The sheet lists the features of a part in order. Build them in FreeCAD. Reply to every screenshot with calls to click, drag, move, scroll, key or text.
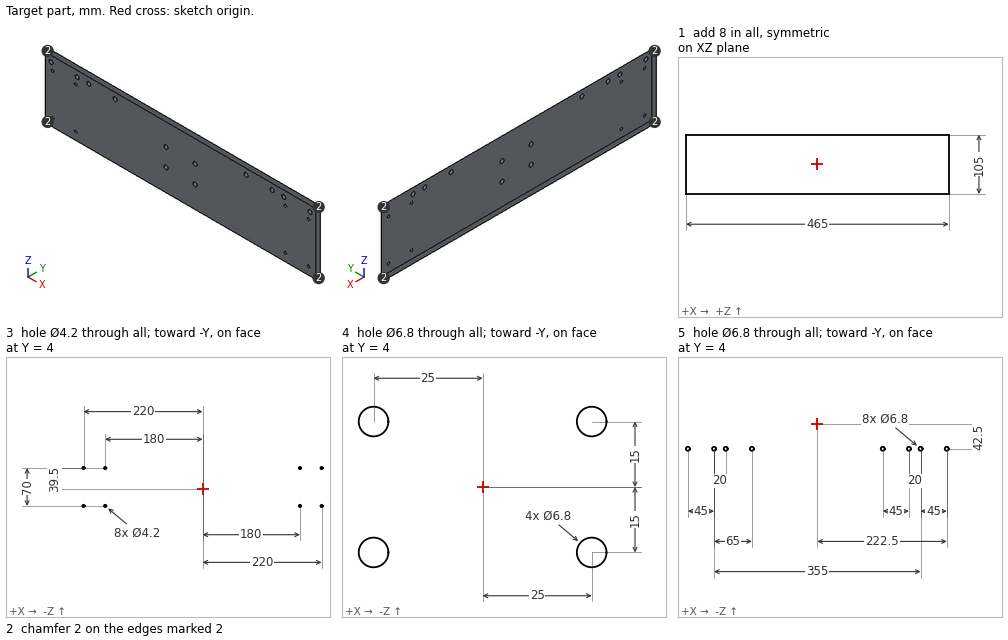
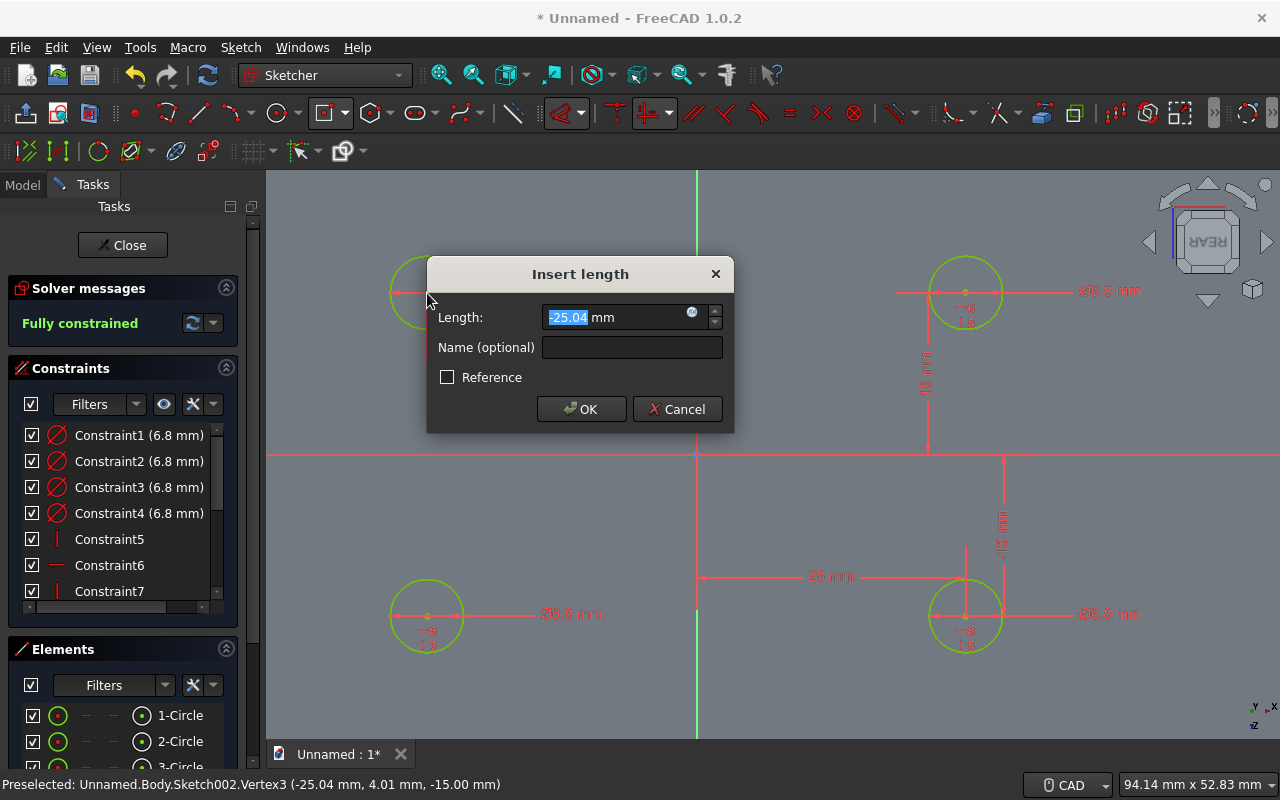
text(-25)
key(Return)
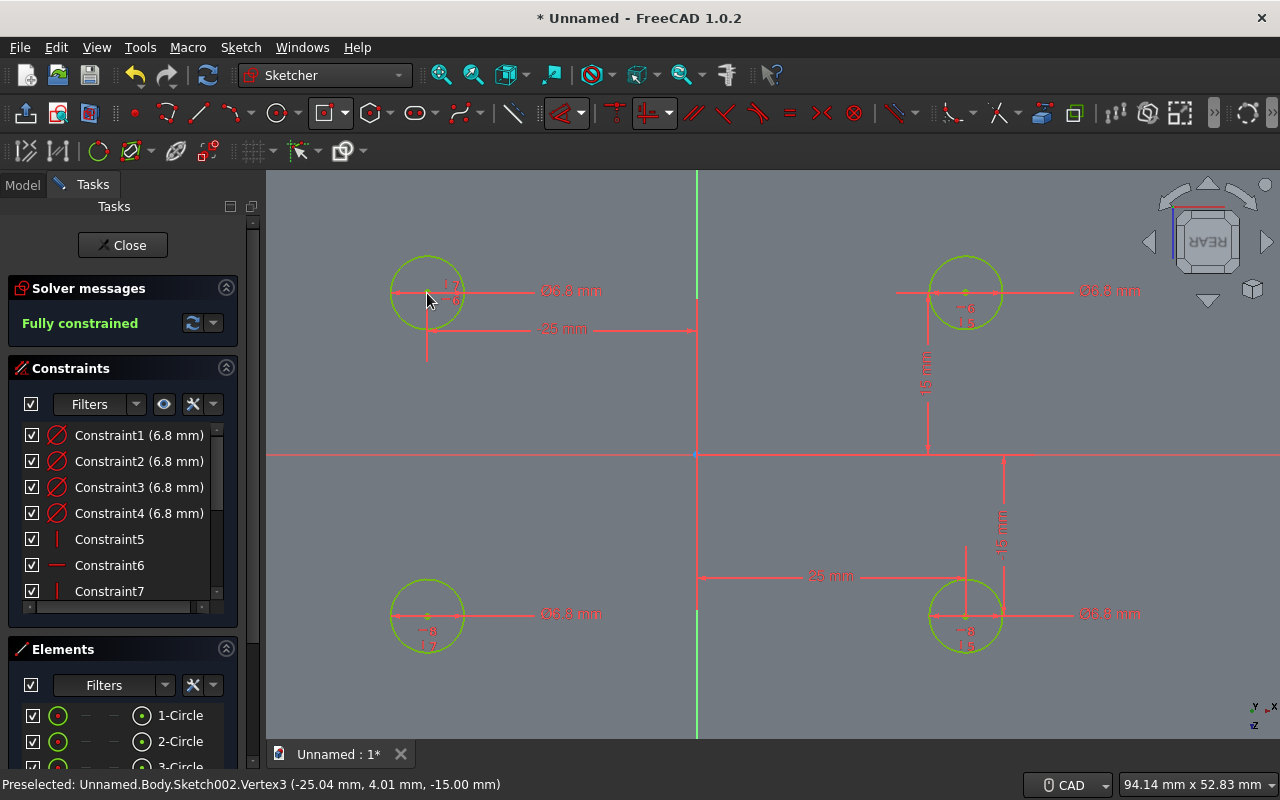
click(123, 245)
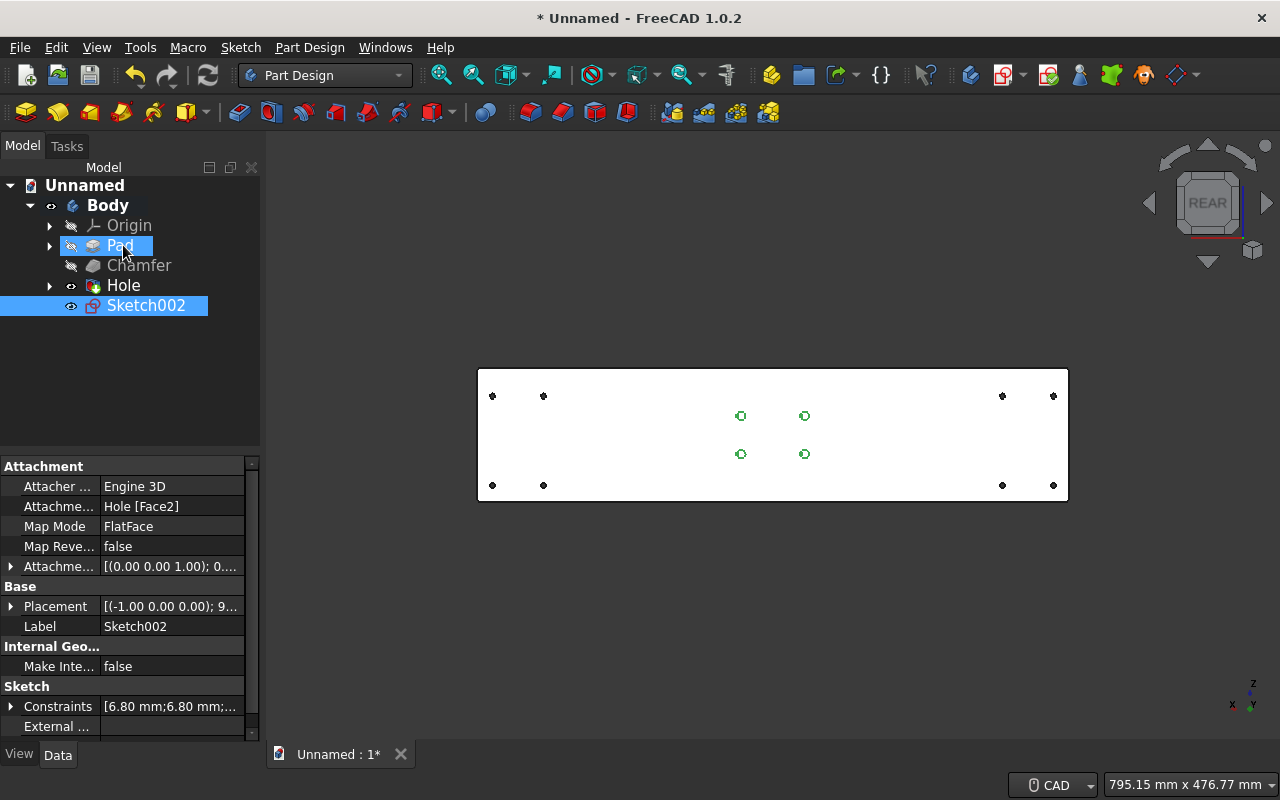
click(272, 112)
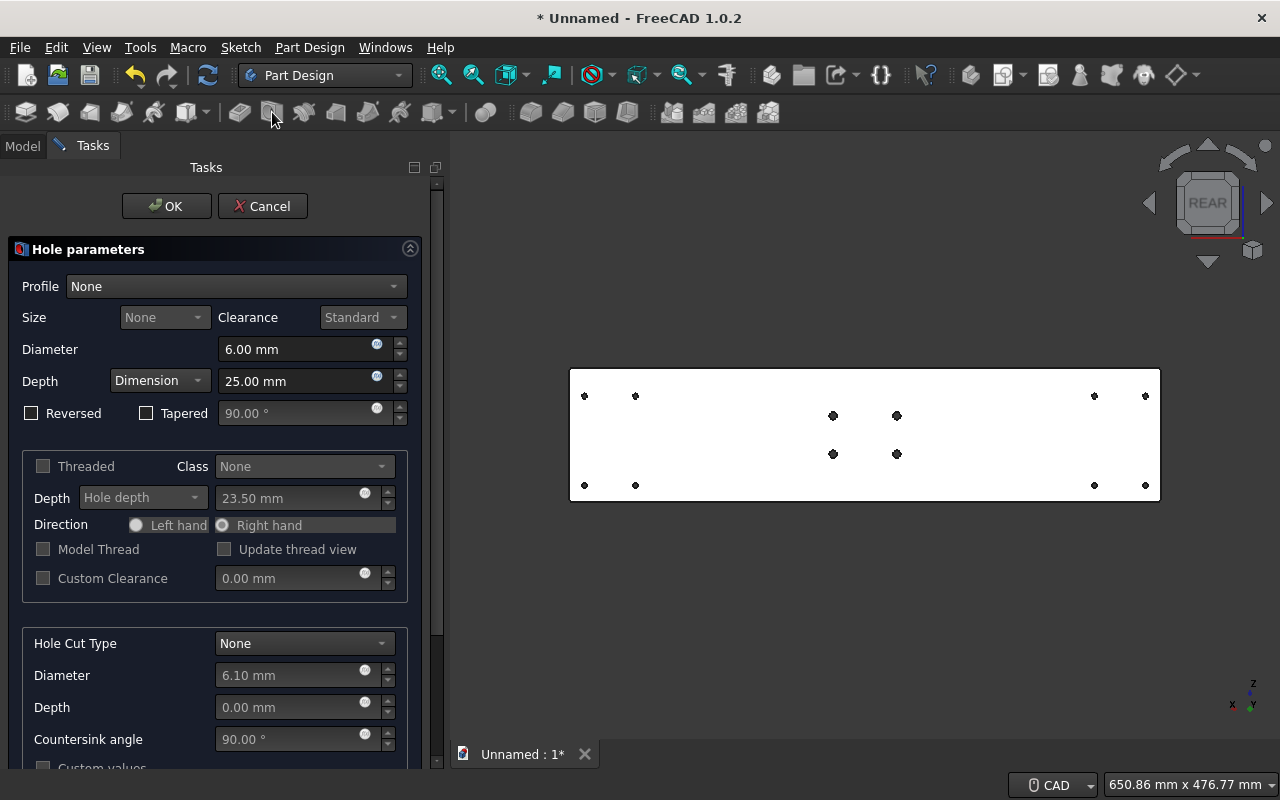
triple_click(305, 349)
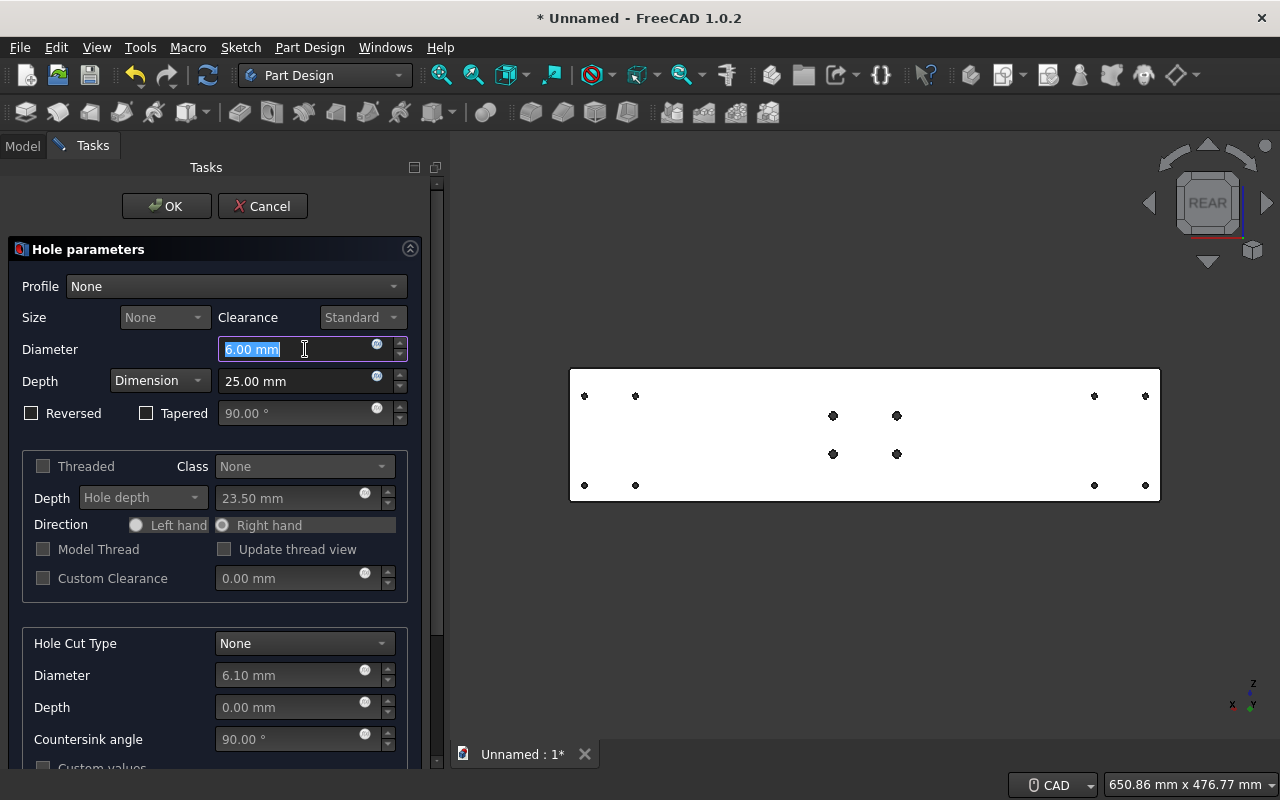
text(6.8)
key(Tab)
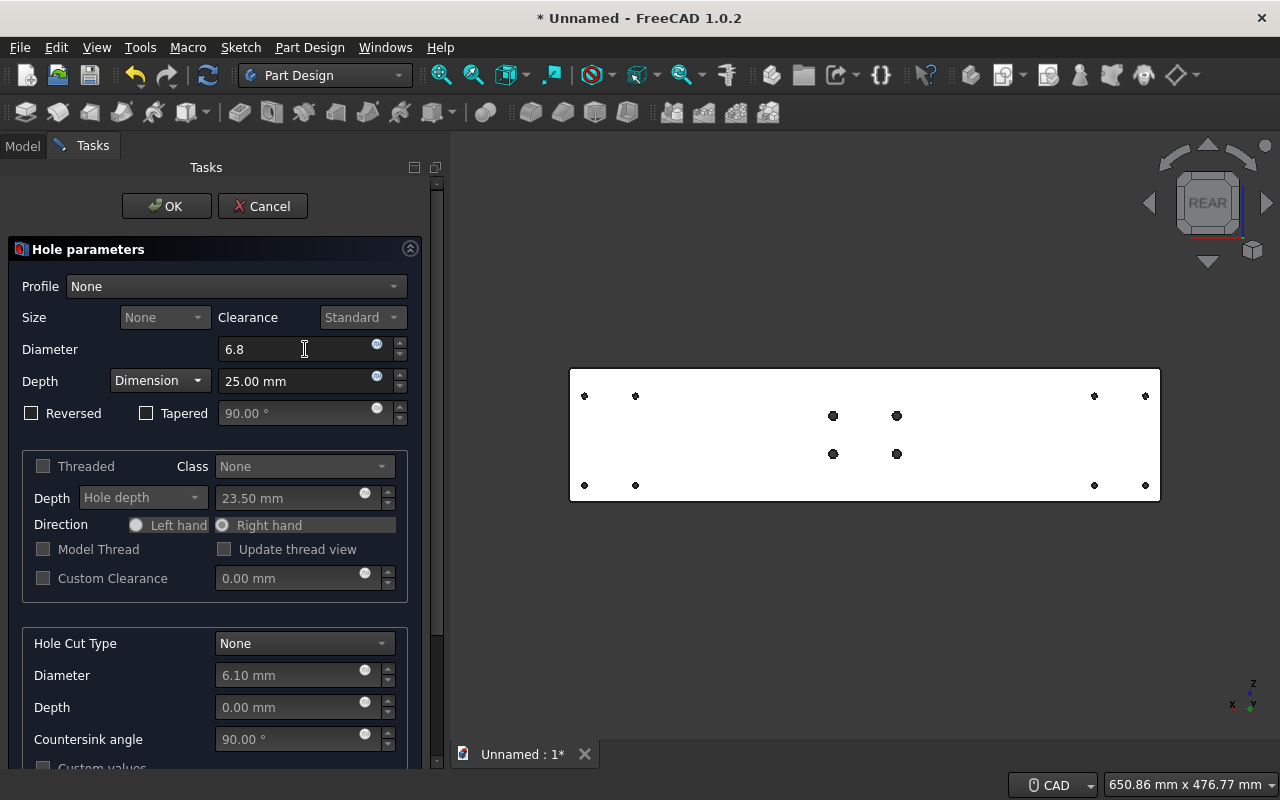
click(161, 380)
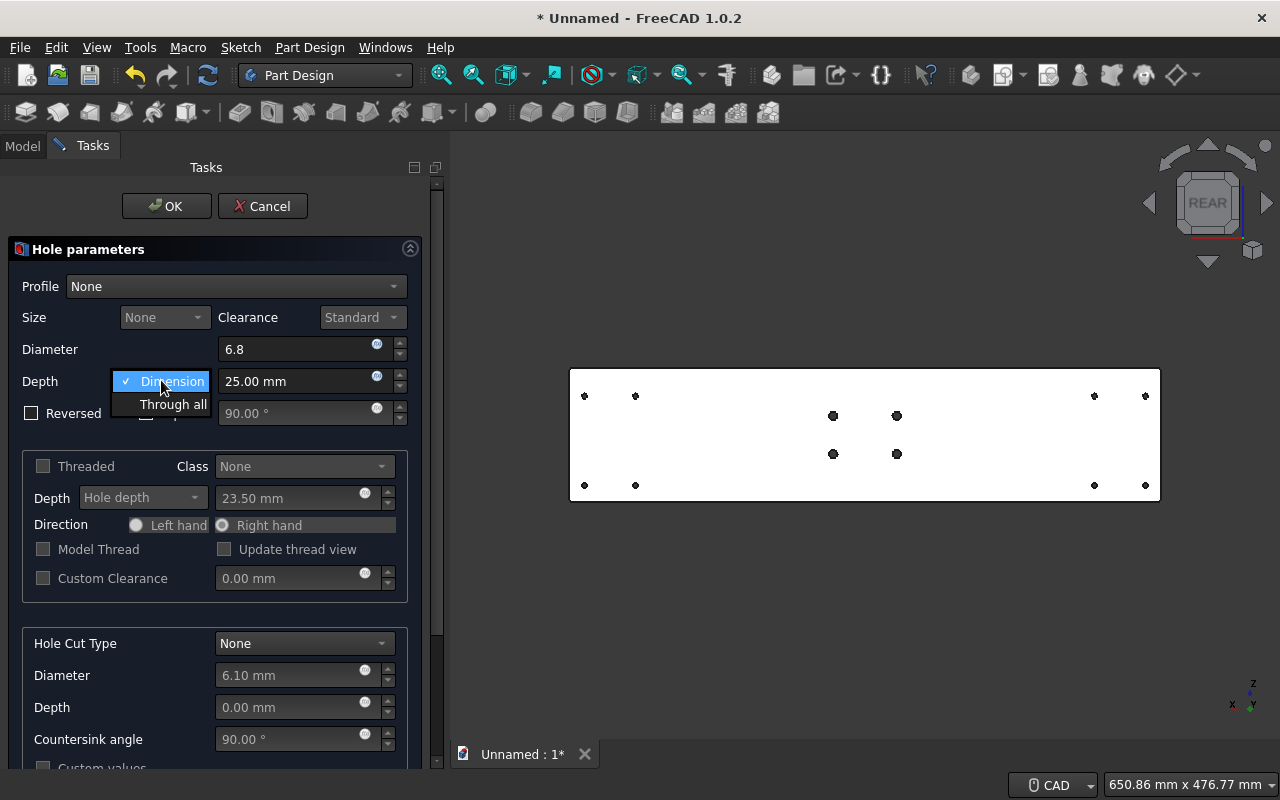
click(160, 404)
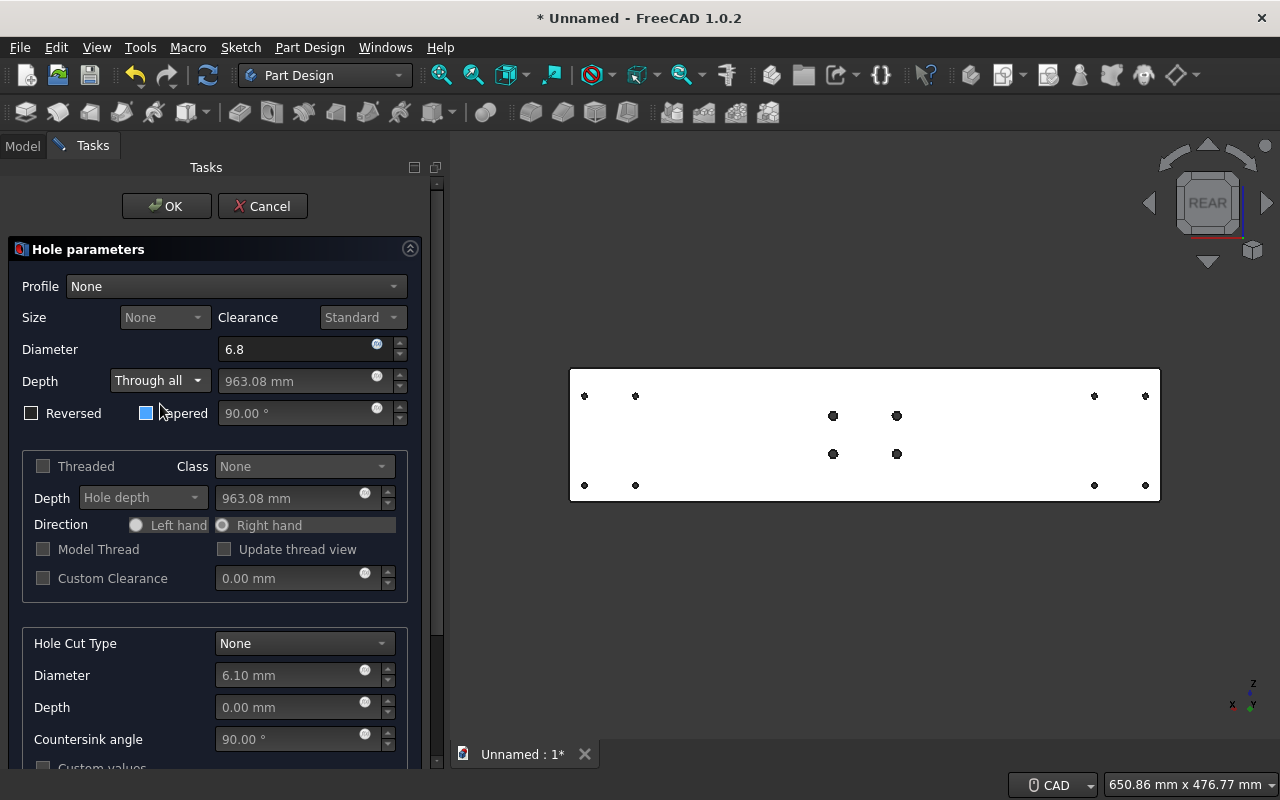
click(167, 206)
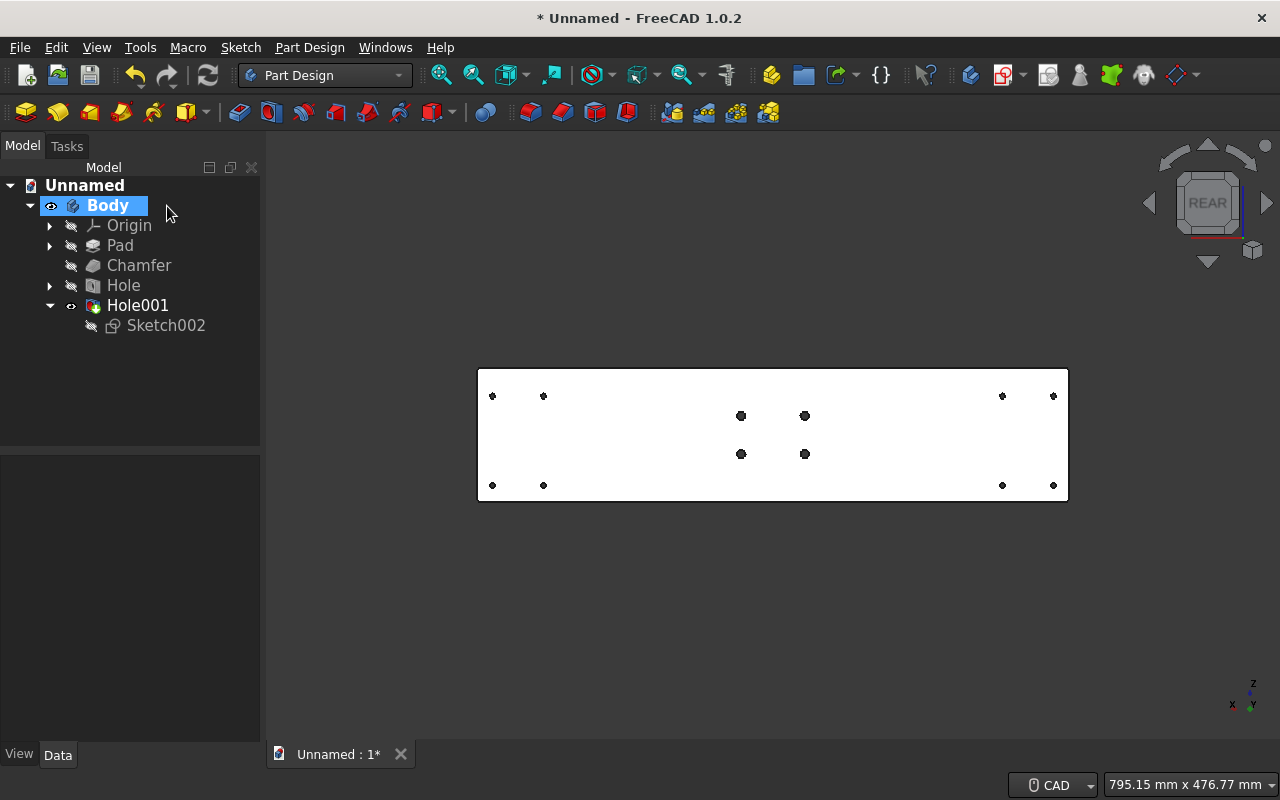
click(604, 434)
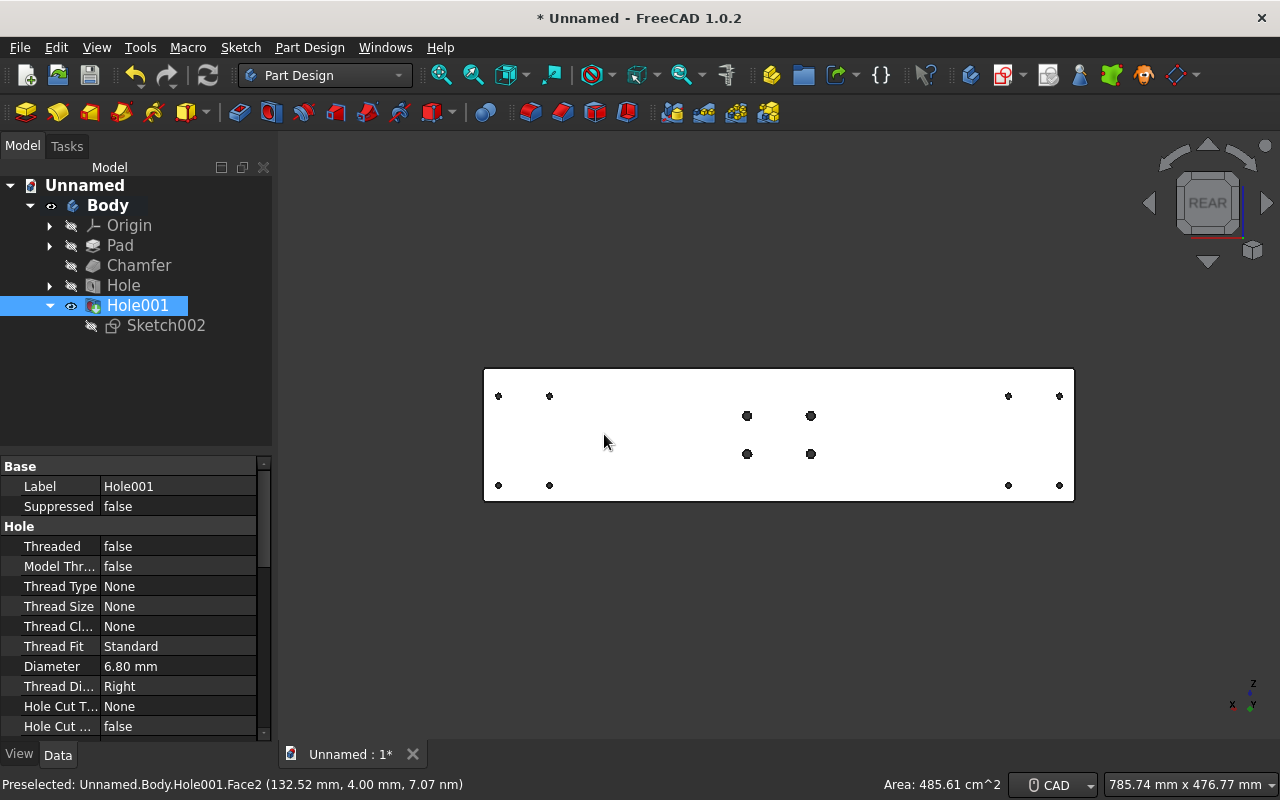
click(1004, 76)